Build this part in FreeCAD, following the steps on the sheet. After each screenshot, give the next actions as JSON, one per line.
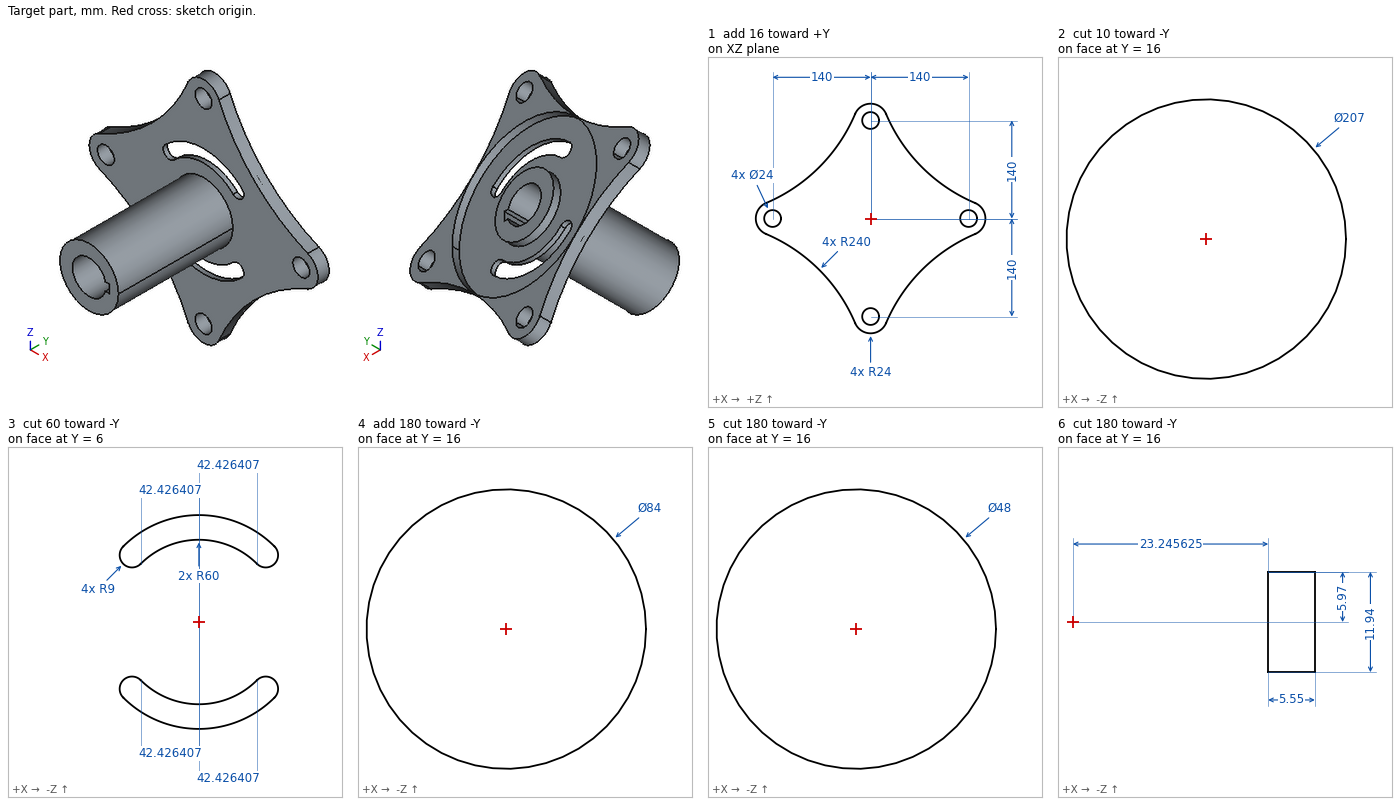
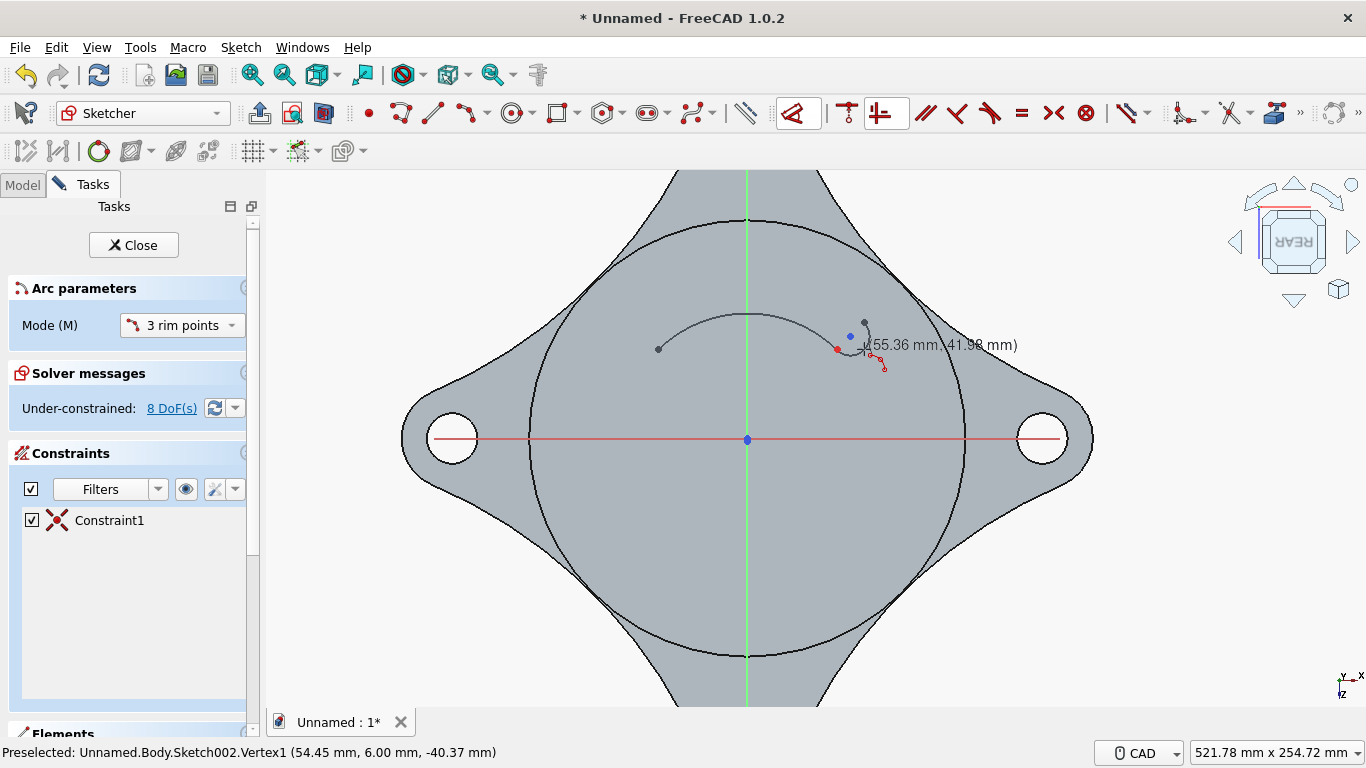
{"action": "left_click", "coordinate": [864, 323]}
{"action": "left_click", "coordinate": [631, 322]}
{"action": "left_click", "coordinate": [773, 276]}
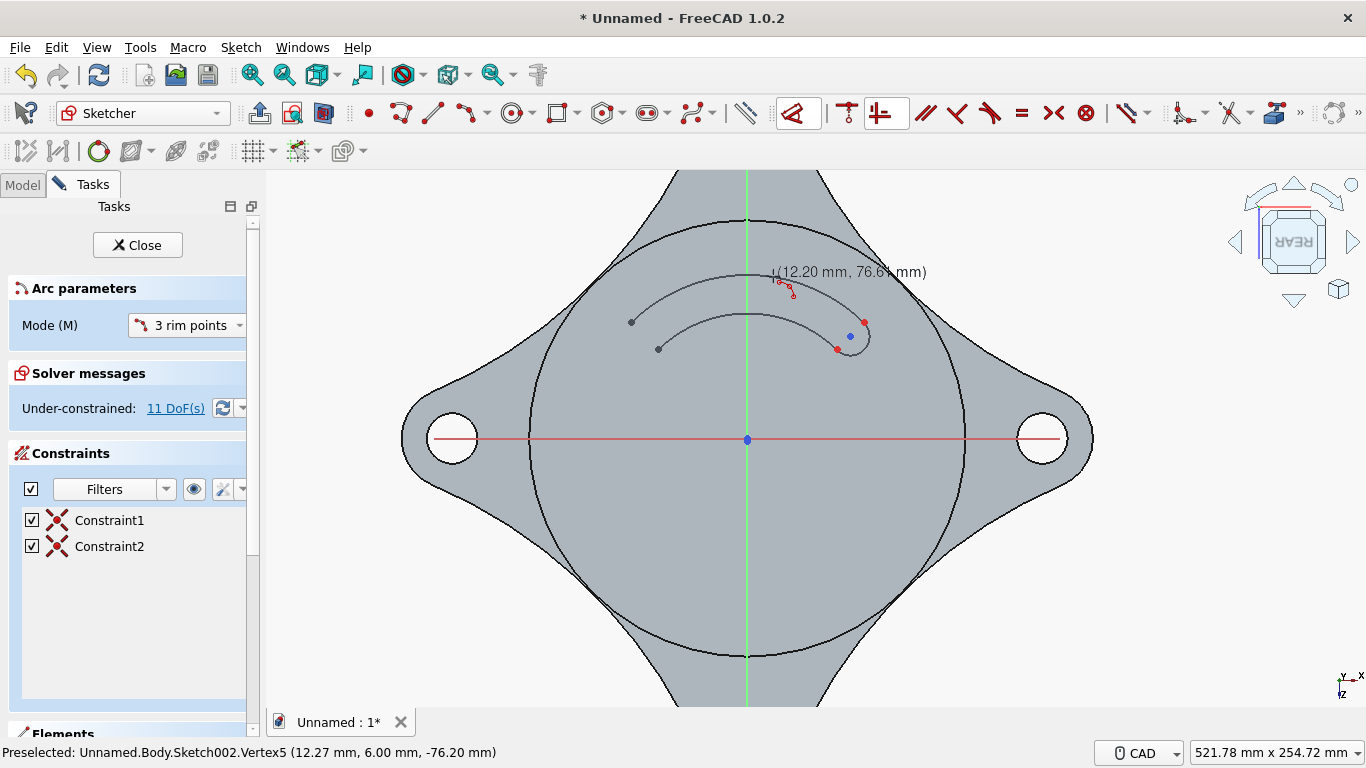
{"action": "left_click", "coordinate": [631, 323]}
{"action": "left_click", "coordinate": [658, 350]}
{"action": "left_click", "coordinate": [631, 349]}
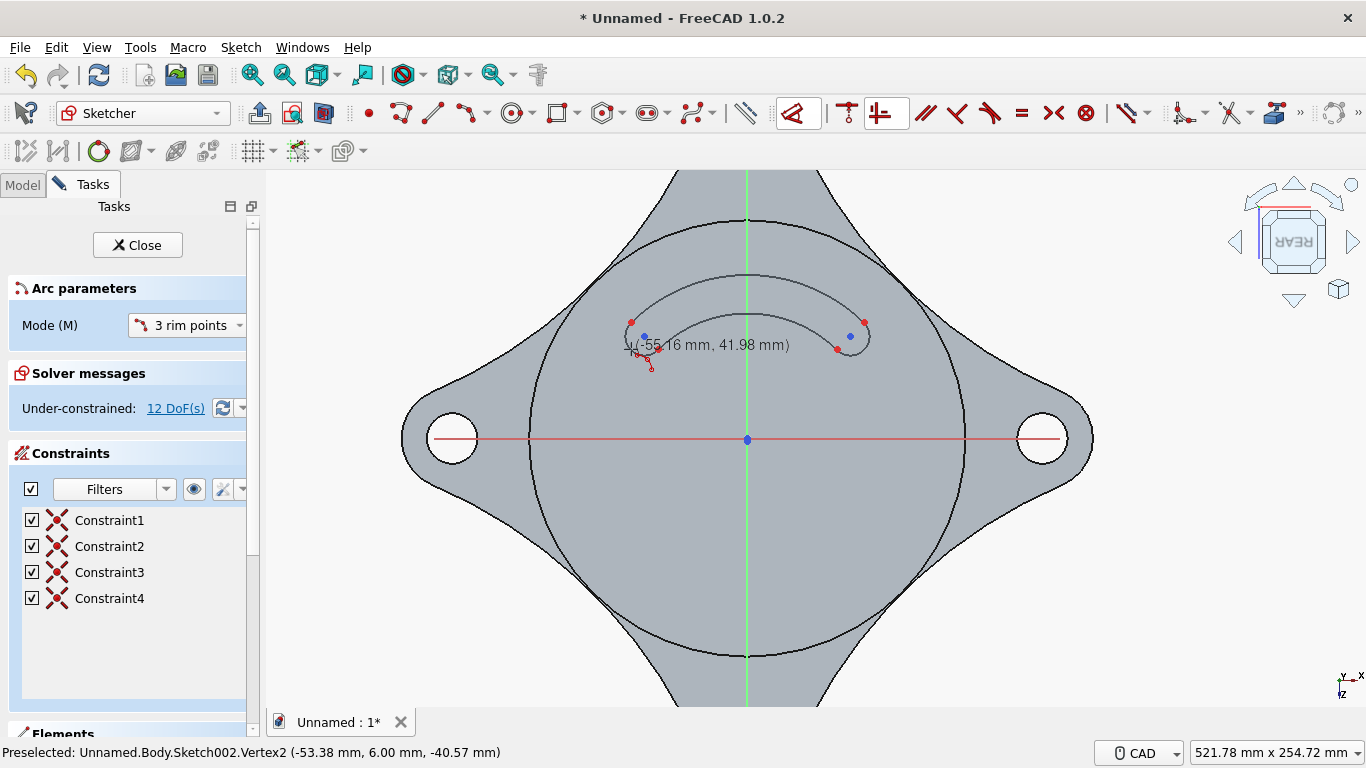
{"action": "left_click", "coordinate": [837, 528]}
{"action": "left_click", "coordinate": [658, 528]}
{"action": "left_click", "coordinate": [728, 563]}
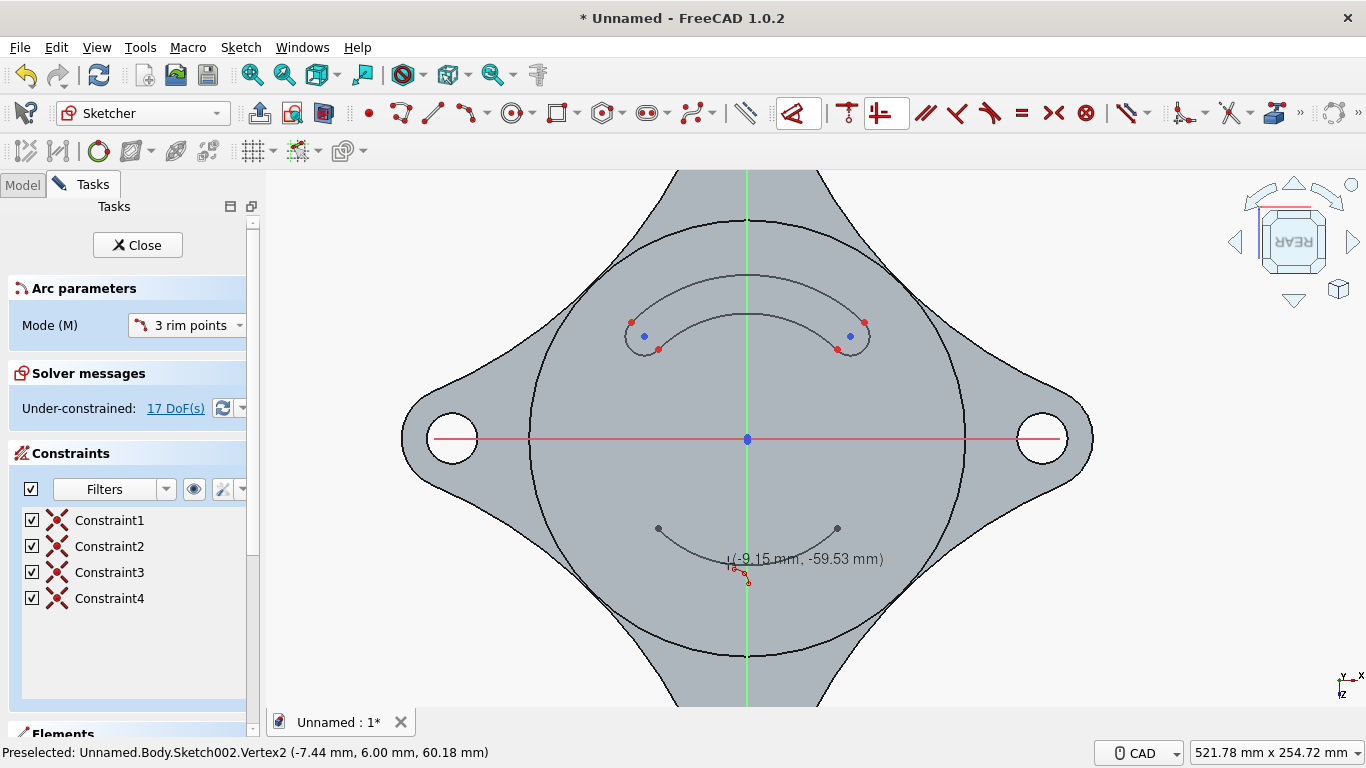
{"action": "left_click", "coordinate": [658, 529]}
{"action": "left_click", "coordinate": [631, 555]}
{"action": "left_click", "coordinate": [631, 528]}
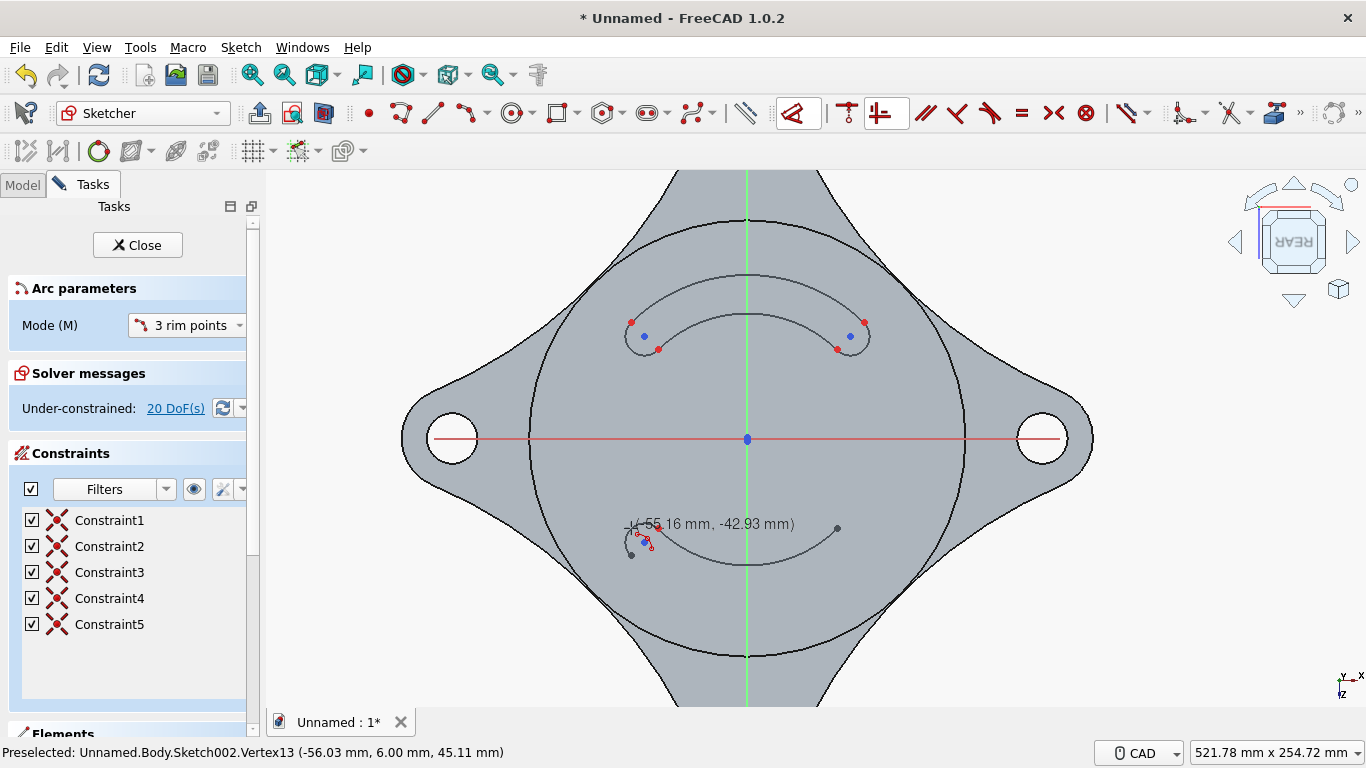
{"action": "left_click", "coordinate": [631, 556]}
{"action": "left_click", "coordinate": [864, 555]}
{"action": "left_click", "coordinate": [722, 601]}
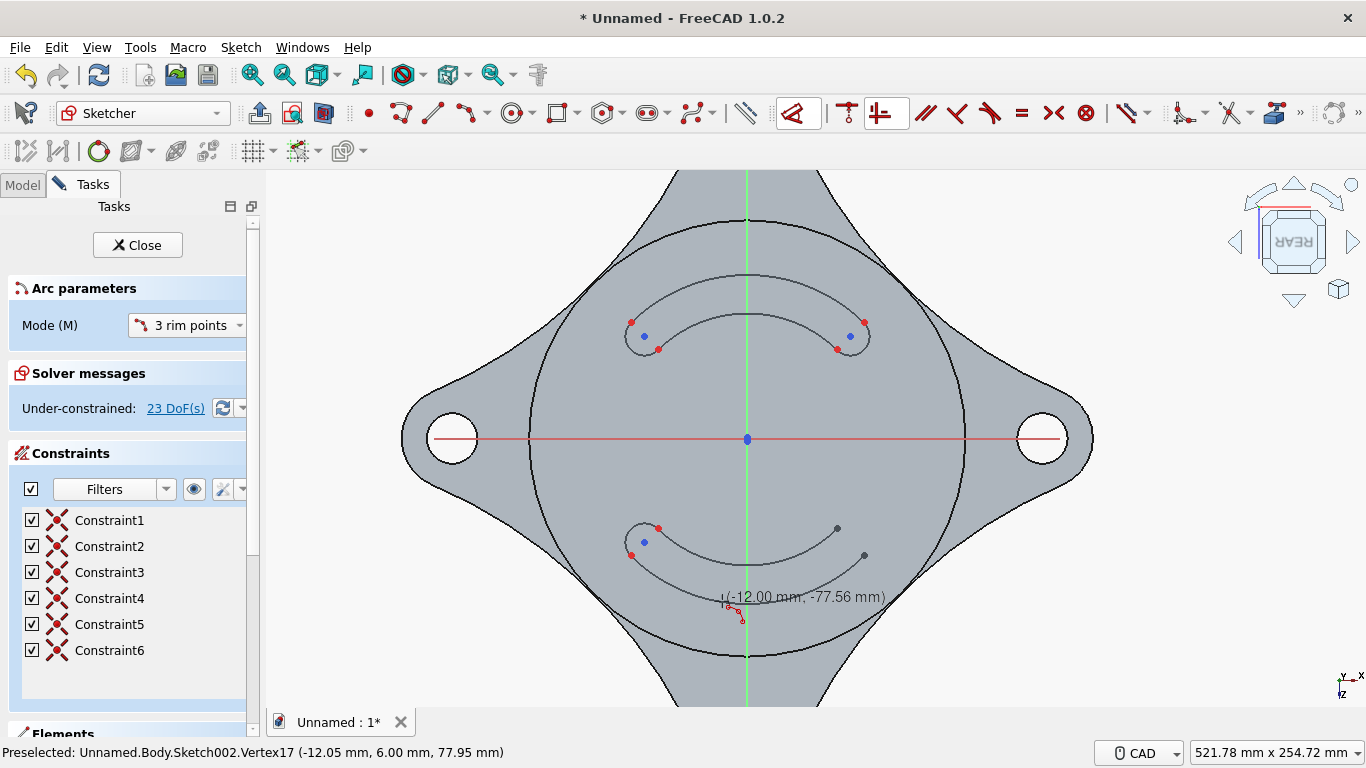
{"action": "left_click", "coordinate": [864, 556]}
{"action": "left_click", "coordinate": [837, 529]}
{"action": "left_click", "coordinate": [864, 528]}
{"action": "key", "text": "Escape"}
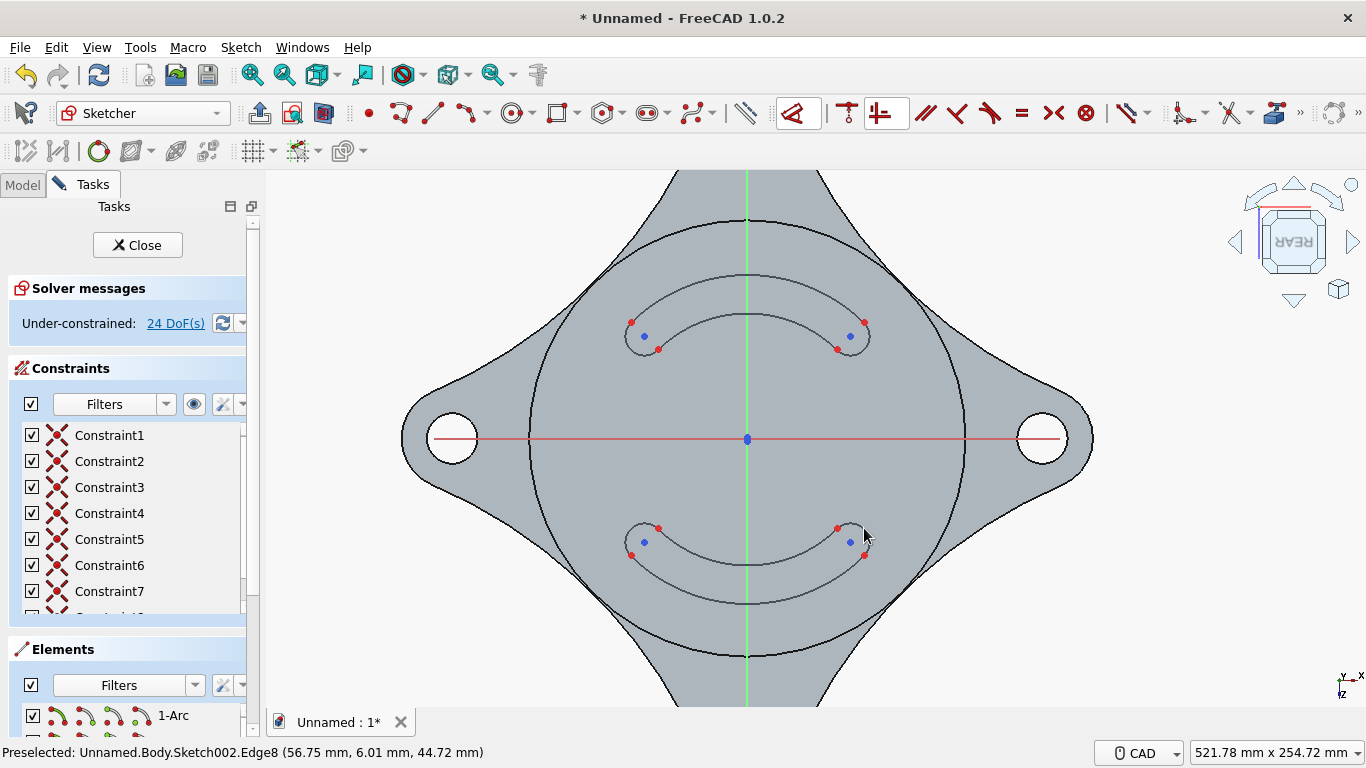
{"action": "left_click", "coordinate": [787, 320]}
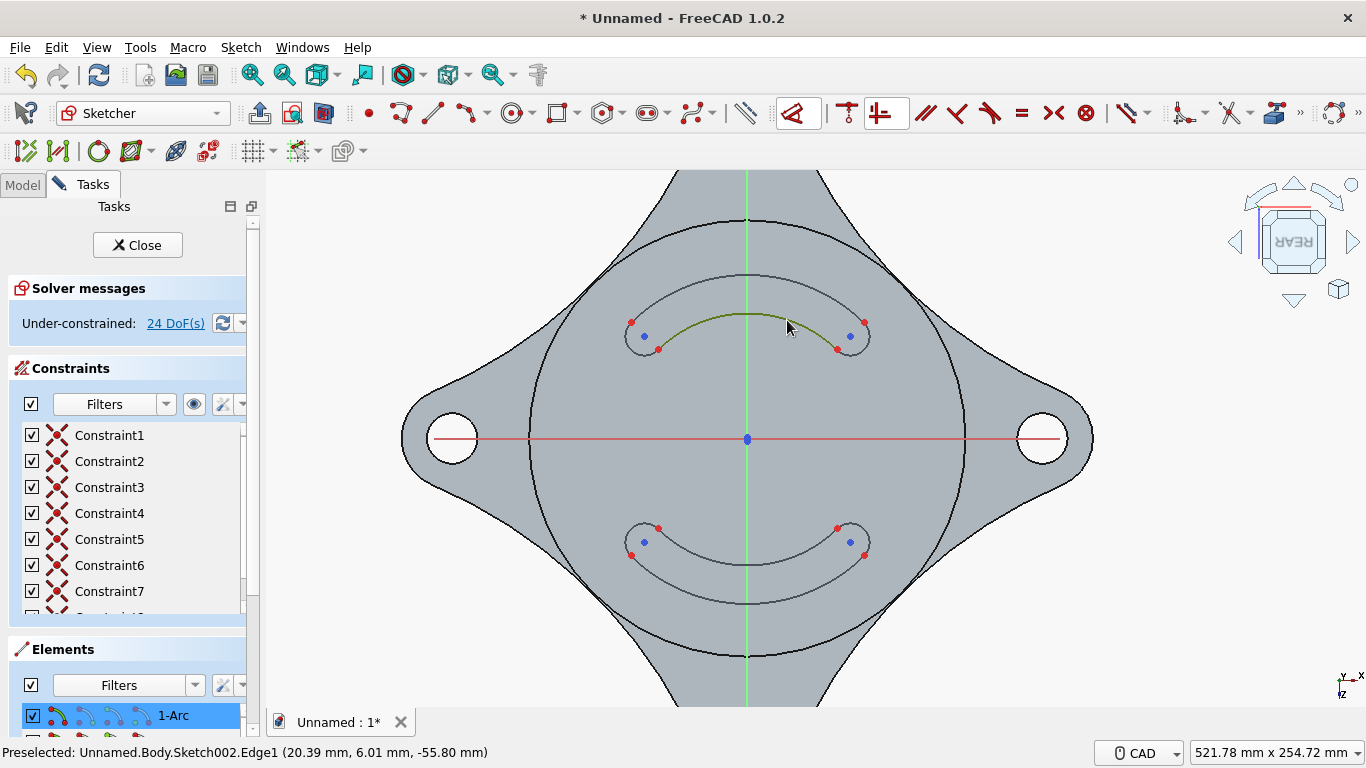
{"action": "left_click", "coordinate": [853, 355]}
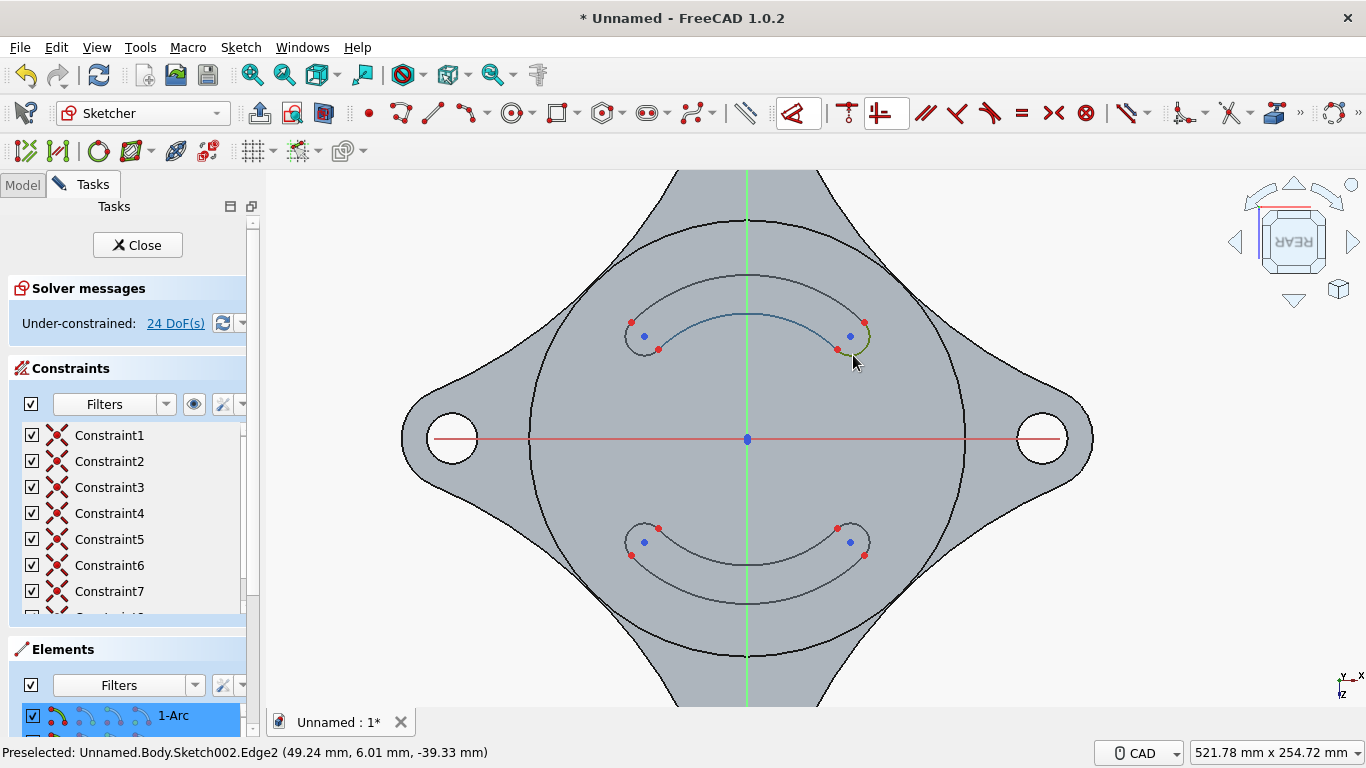
{"action": "left_click", "coordinate": [990, 114]}